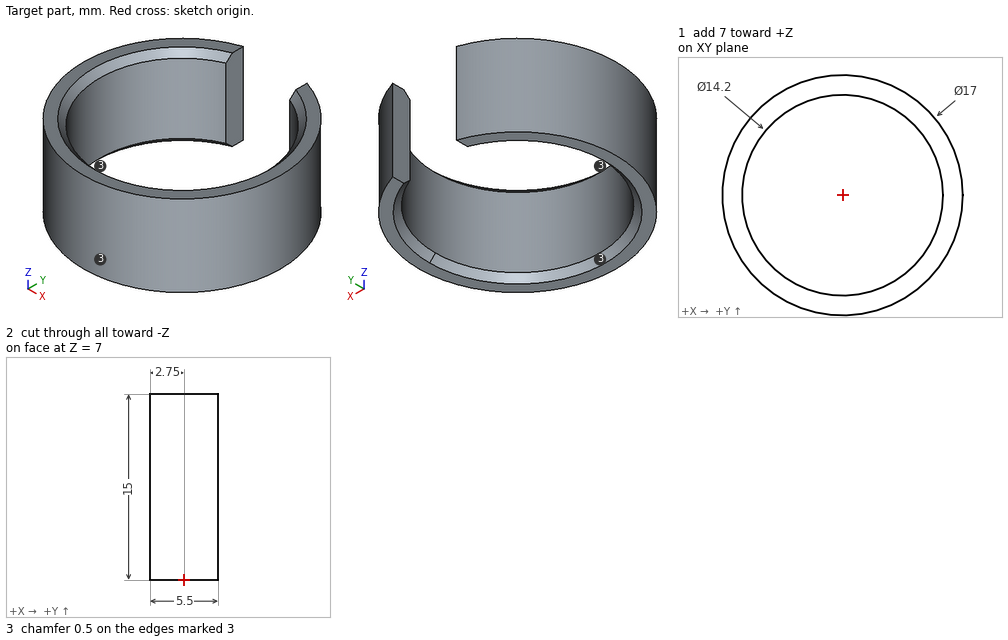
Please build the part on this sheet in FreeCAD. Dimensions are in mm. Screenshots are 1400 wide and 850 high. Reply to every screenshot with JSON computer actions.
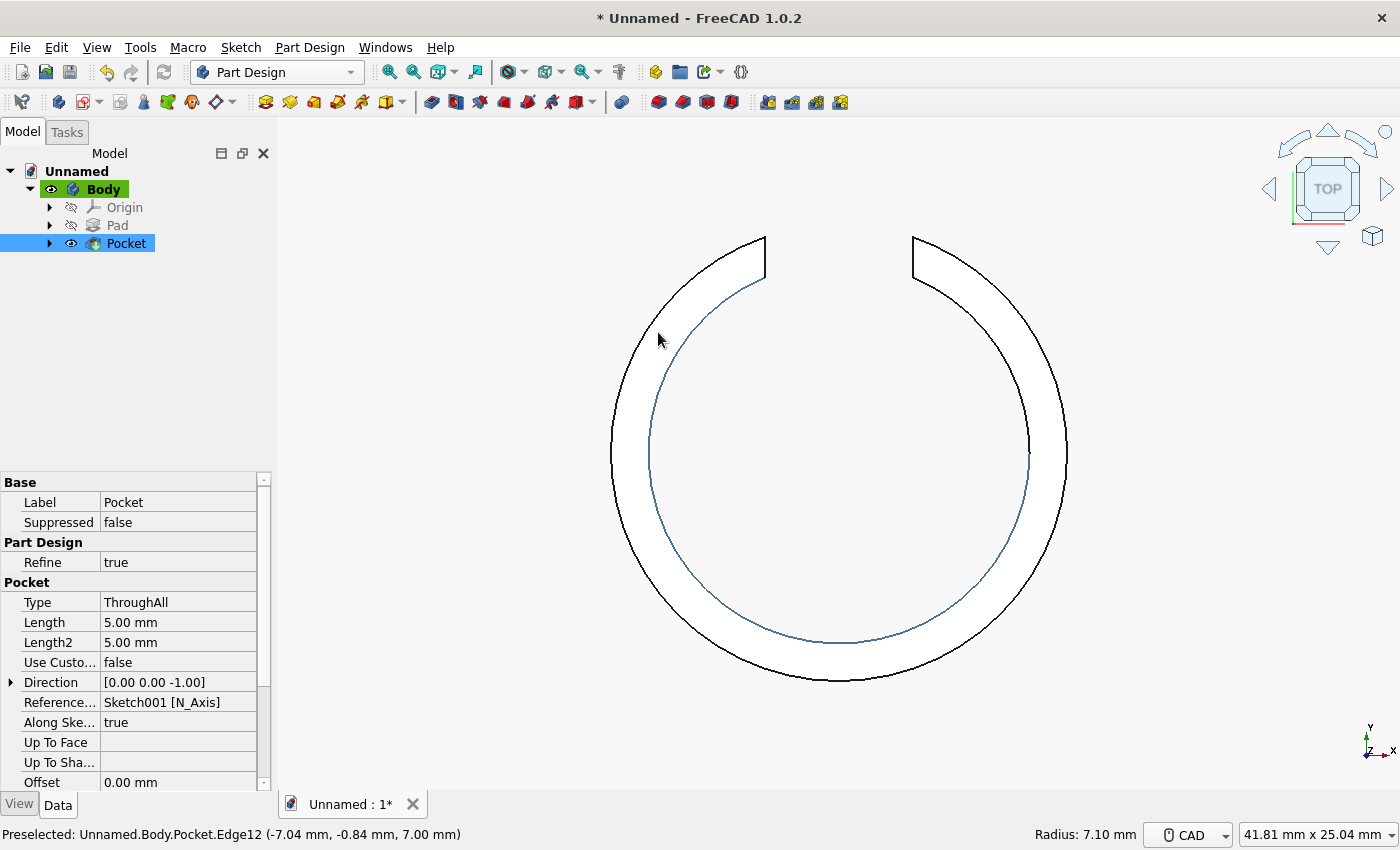
{"action": "key", "text": "1"}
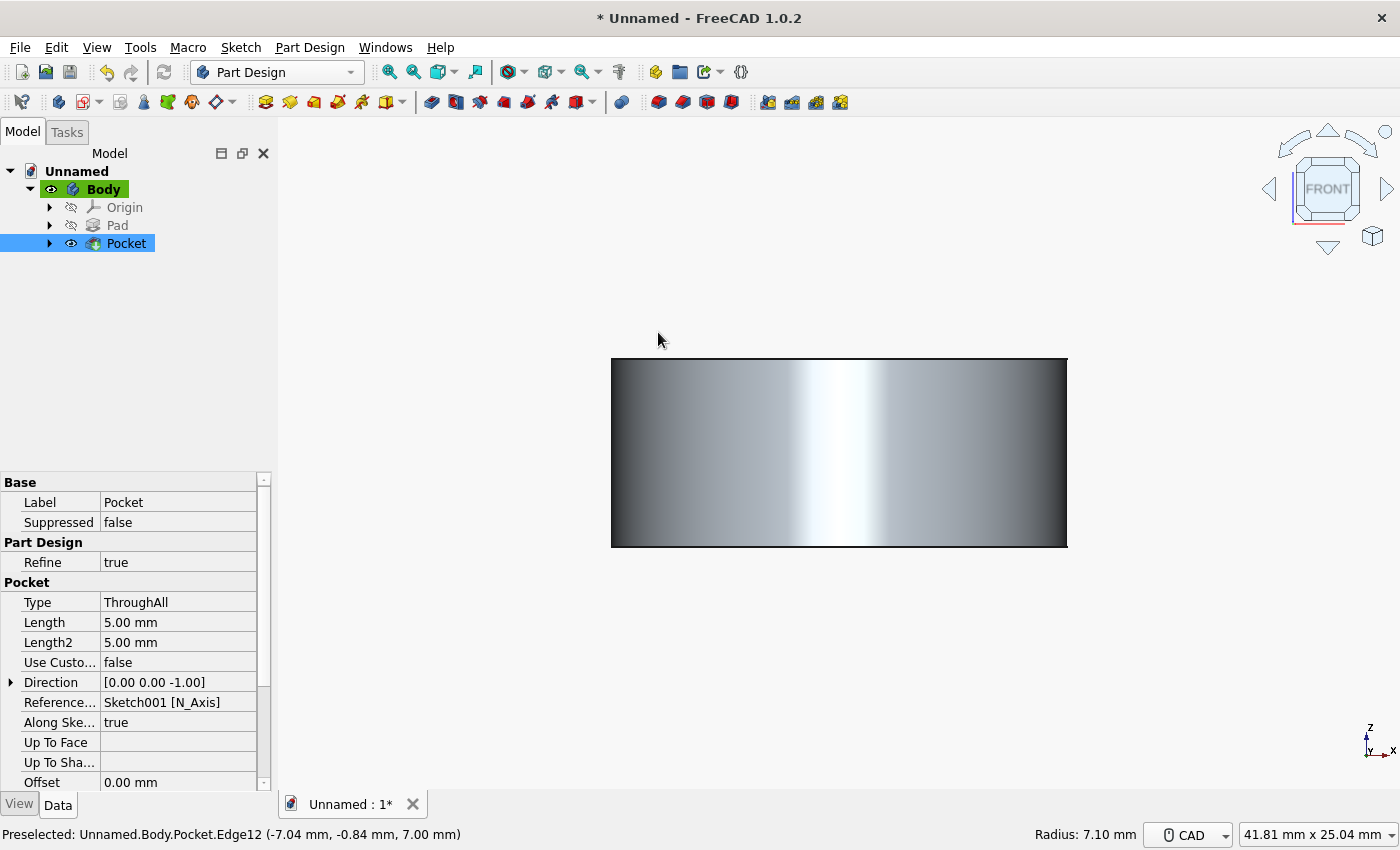
{"action": "left_click", "coordinate": [390, 72]}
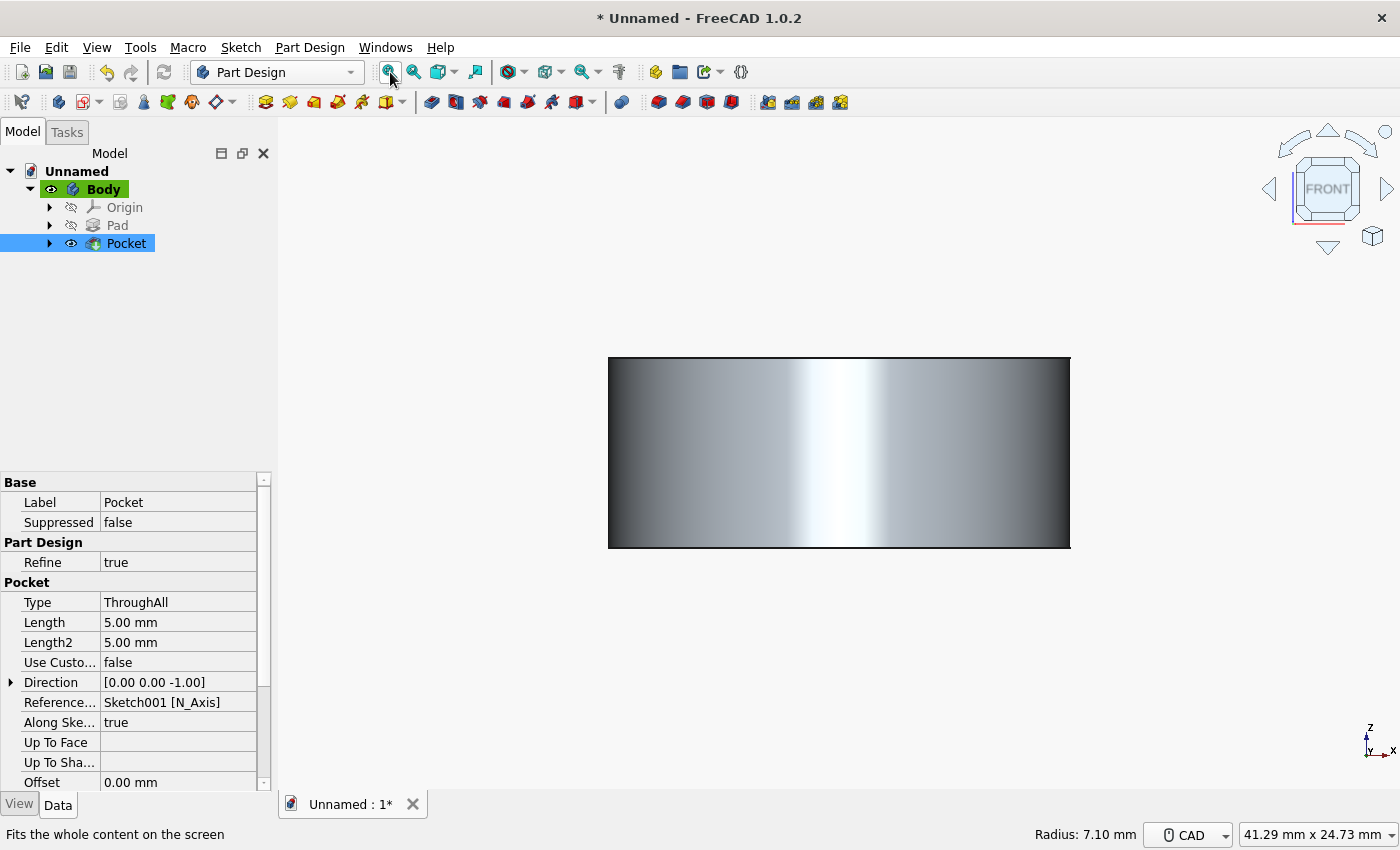
{"action": "key", "text": "3"}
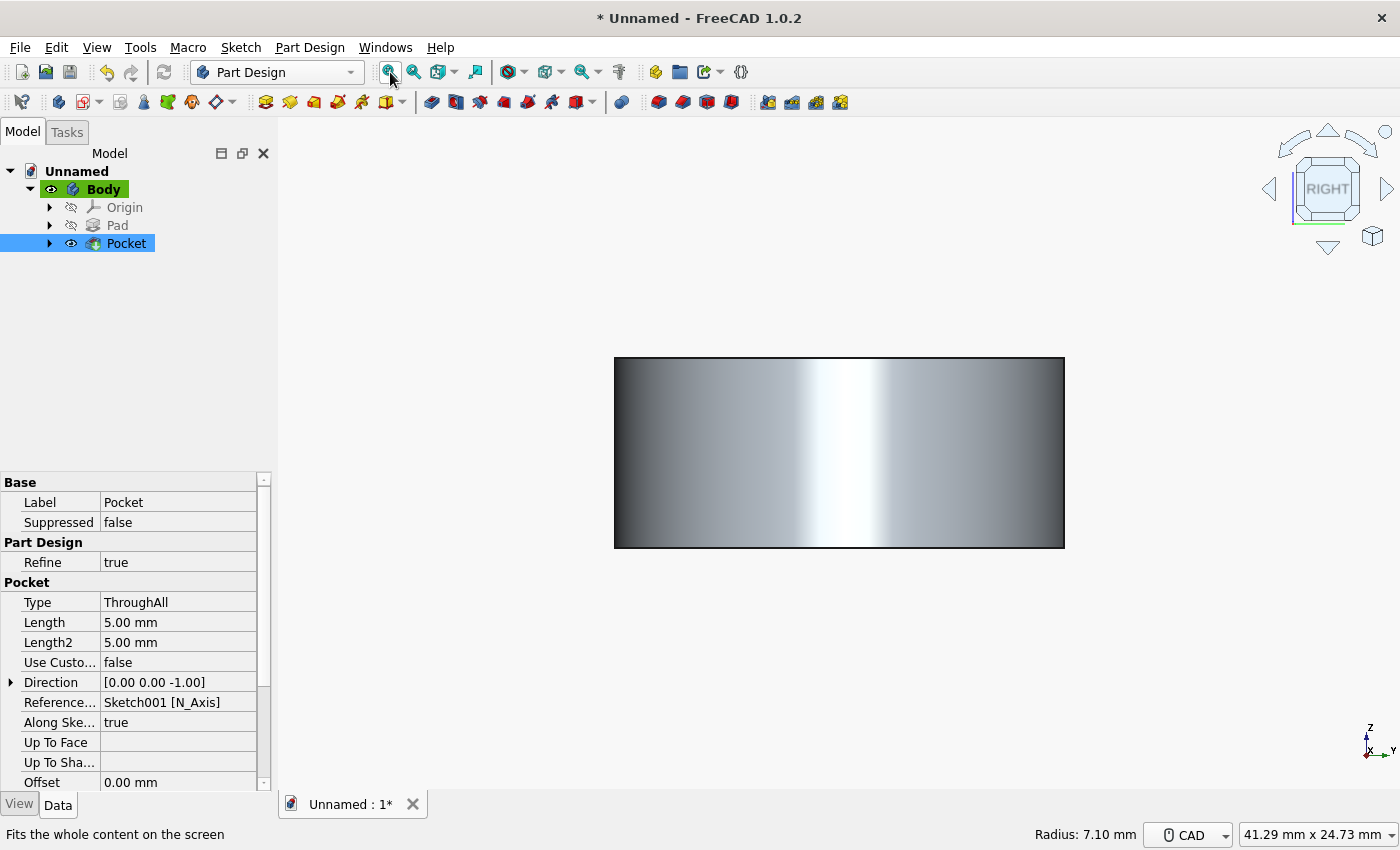
{"action": "left_click", "coordinate": [390, 72]}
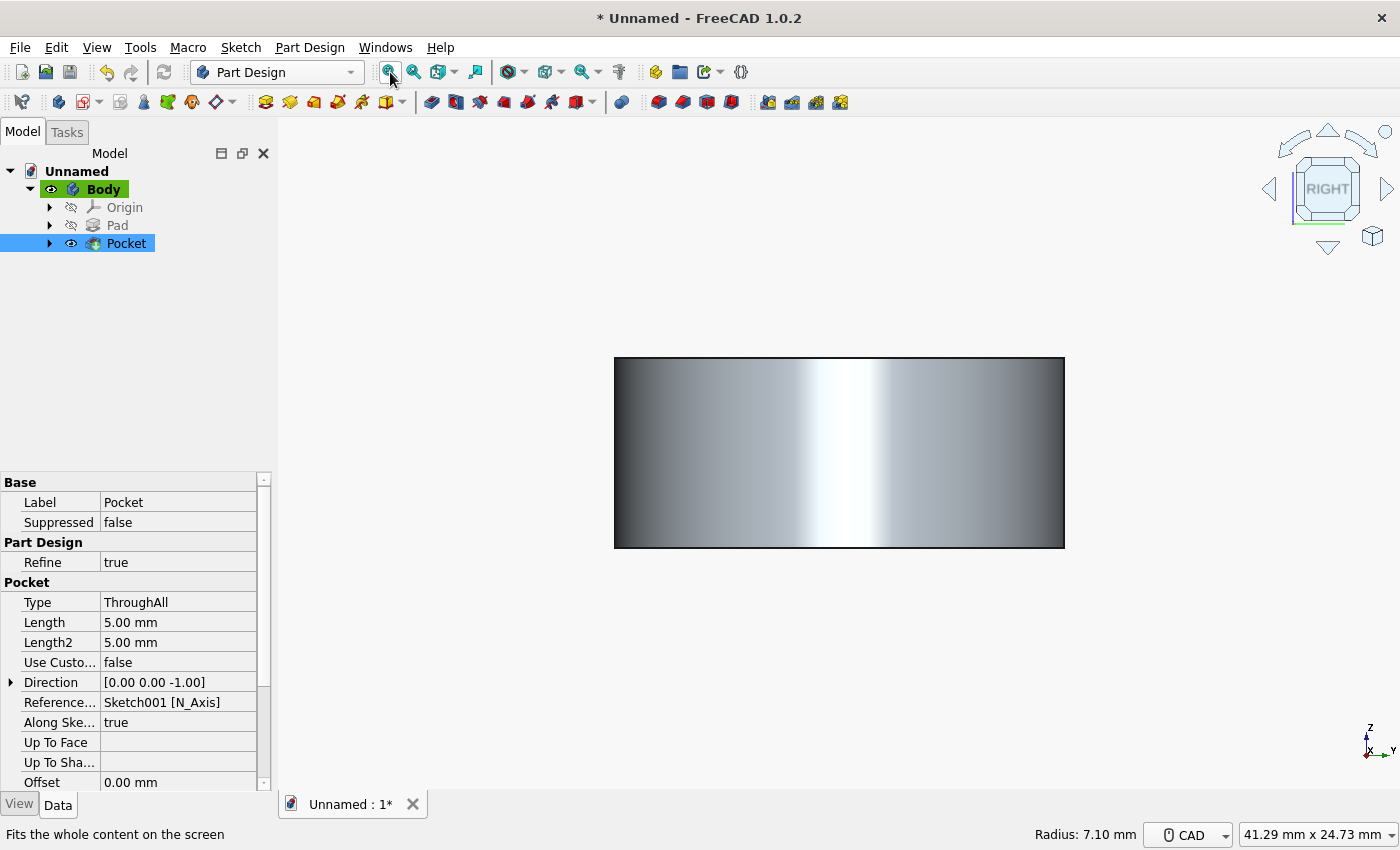
{"action": "key", "text": "5"}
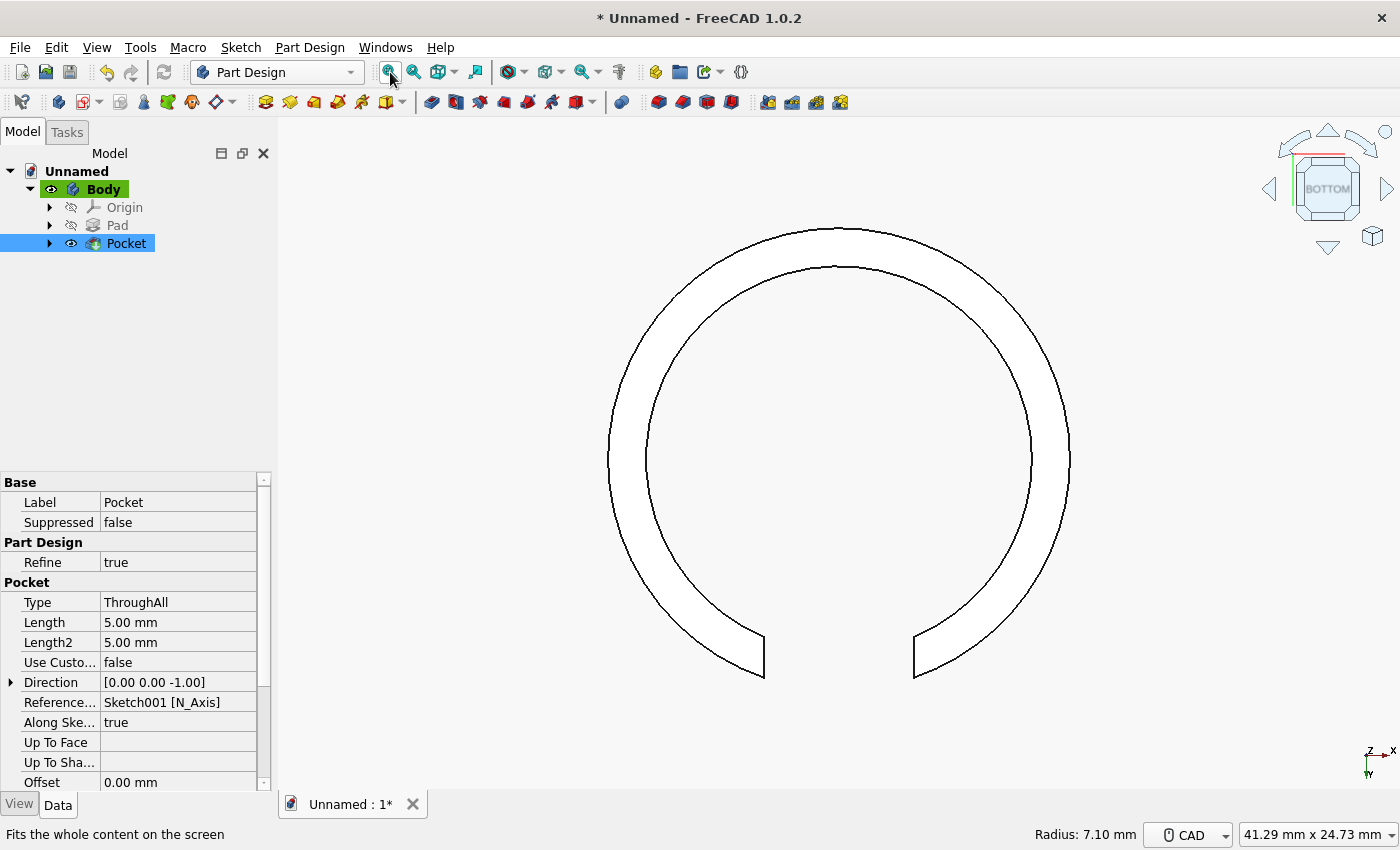
{"action": "left_click", "coordinate": [732, 298], "text": "ctrl"}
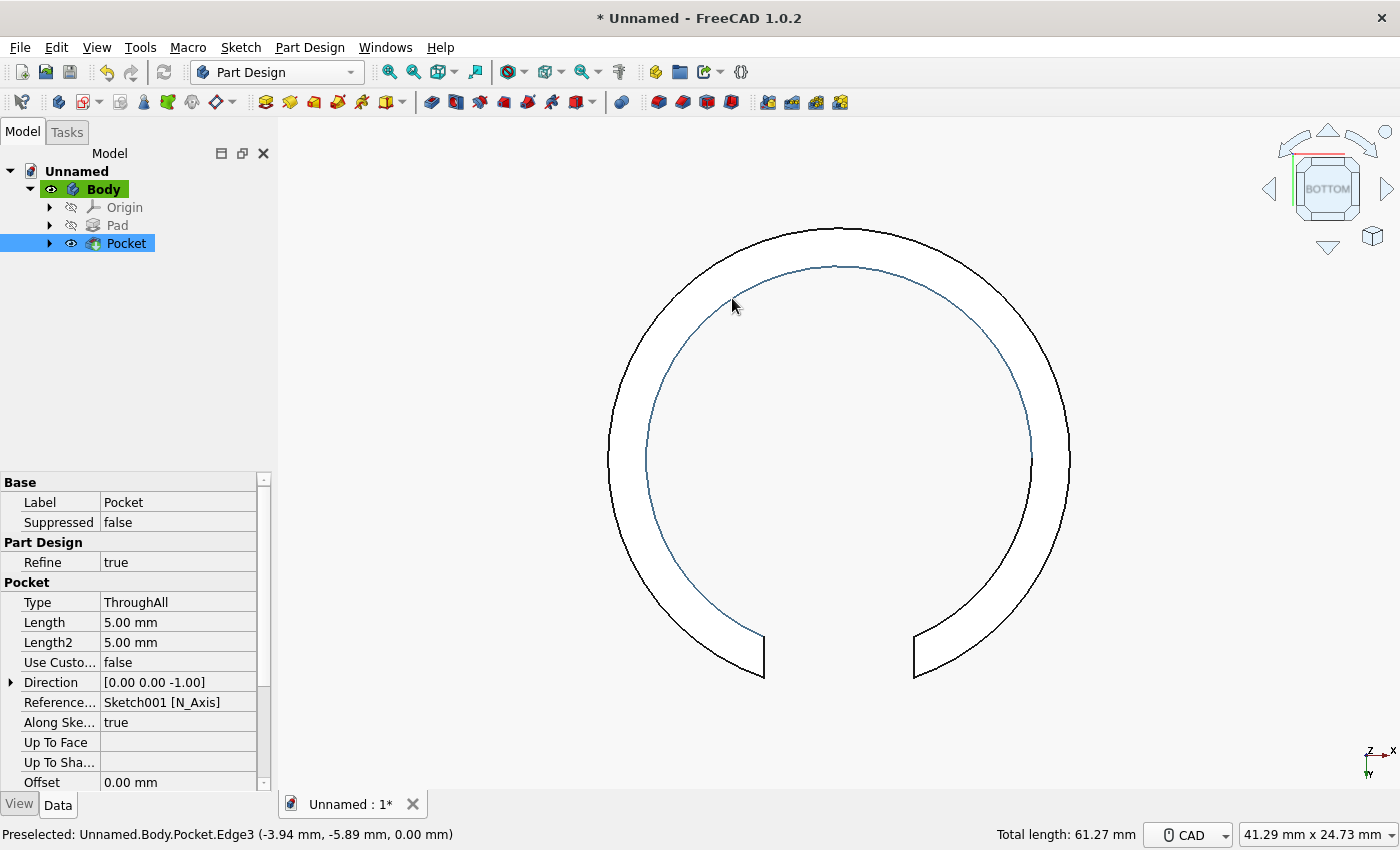
{"action": "left_click", "coordinate": [684, 102]}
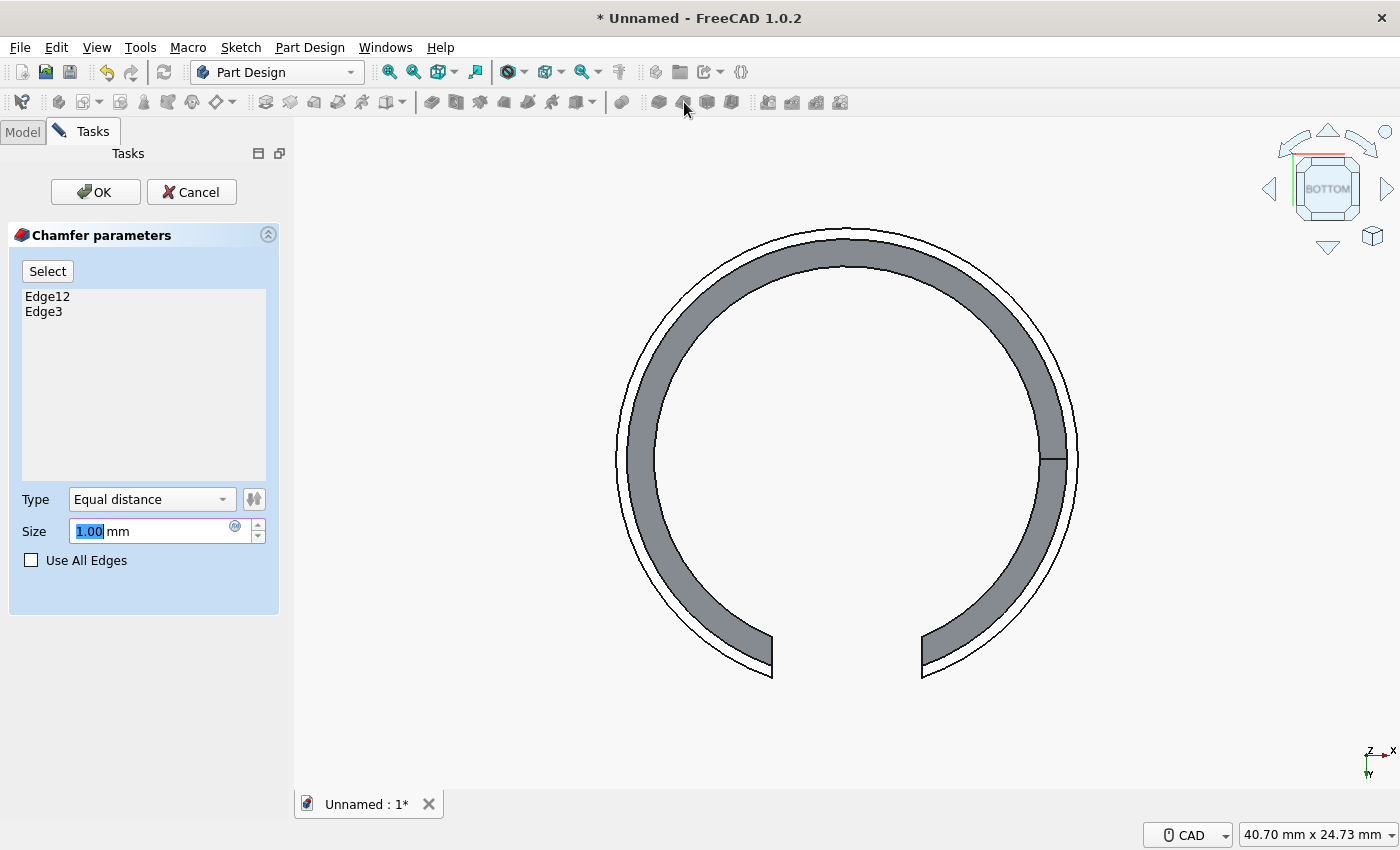
{"action": "type", "text": "0.5"}
{"action": "key", "text": "Tab"}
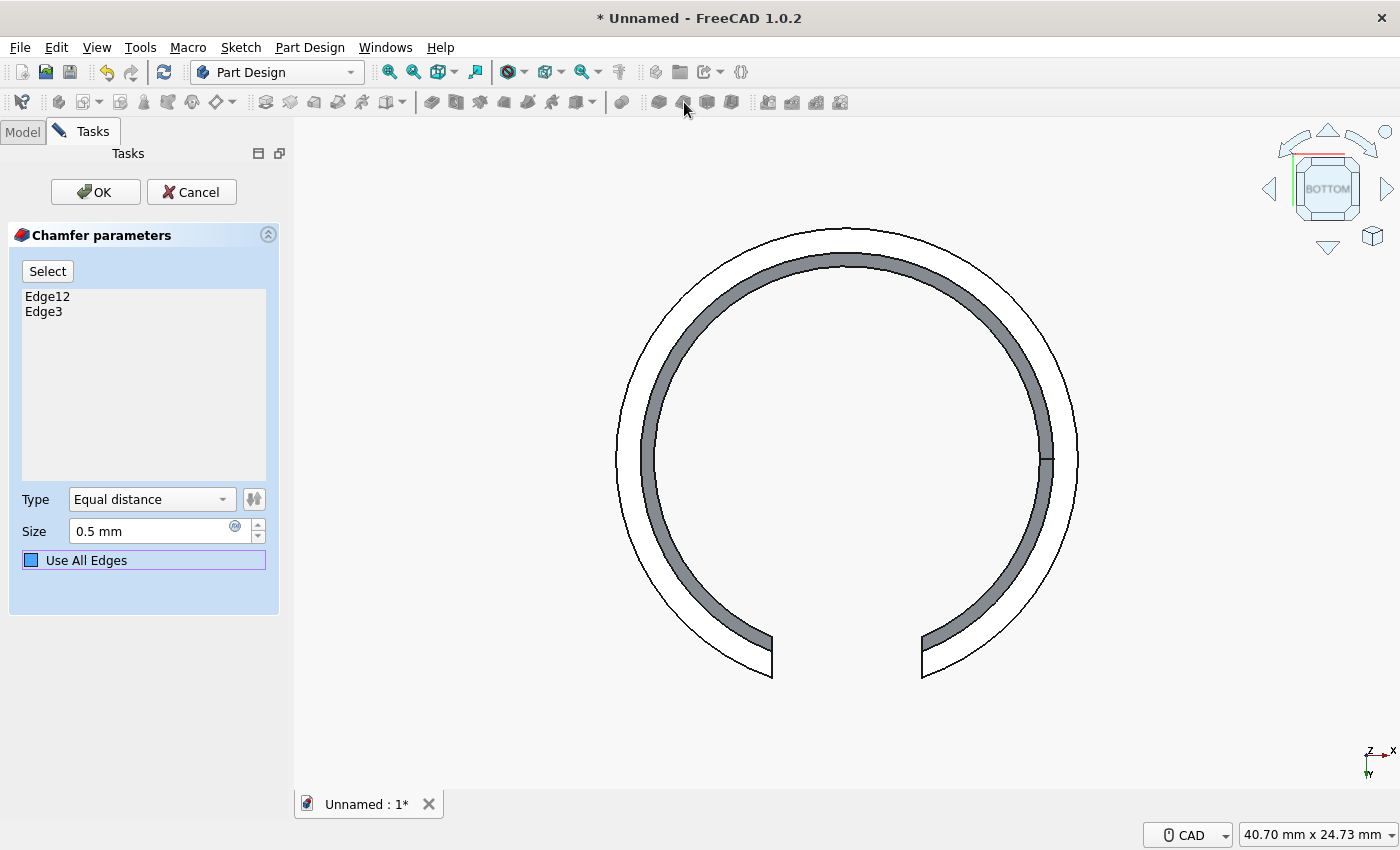
{"action": "left_click", "coordinate": [96, 192]}